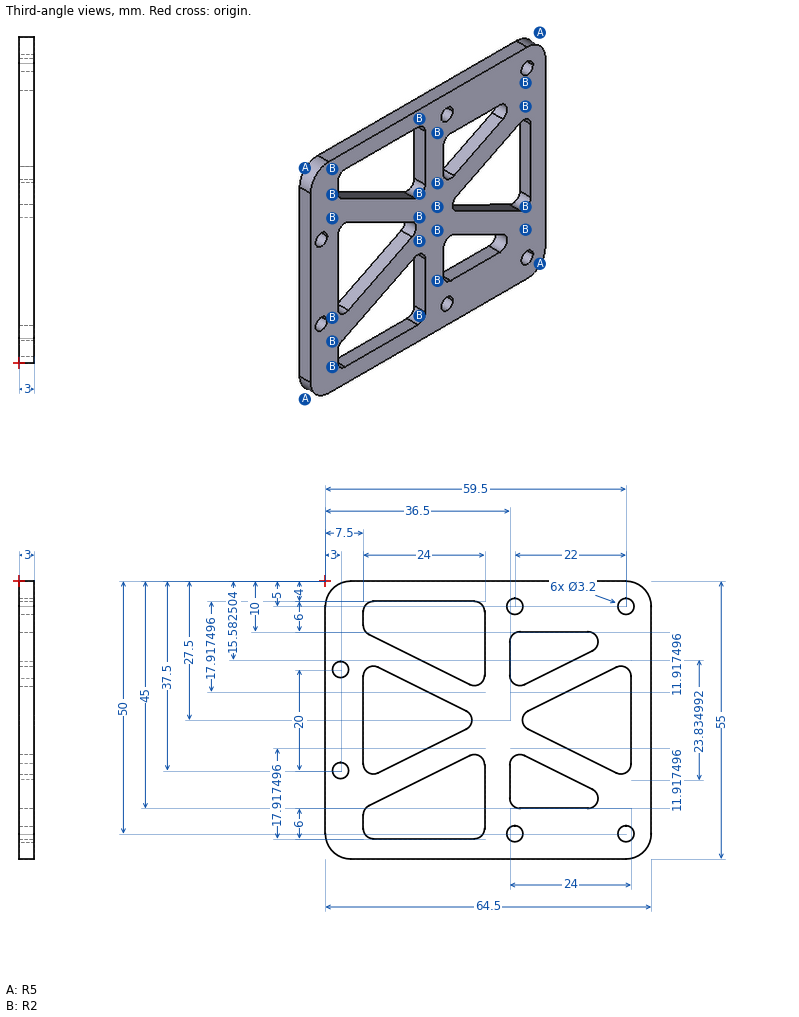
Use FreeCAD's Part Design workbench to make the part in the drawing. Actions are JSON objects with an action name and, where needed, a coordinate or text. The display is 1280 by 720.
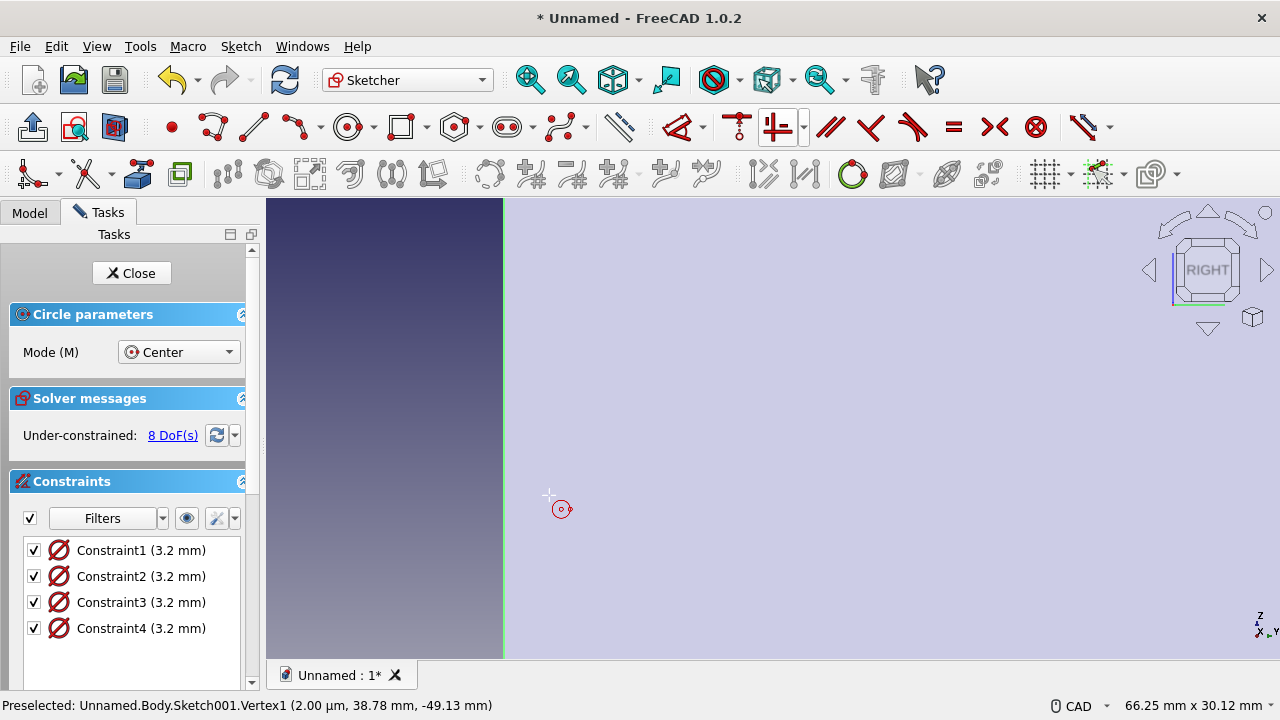
{"action": "left_click", "coordinate": [550, 494]}
{"action": "mouse_move", "coordinate": [567, 477]}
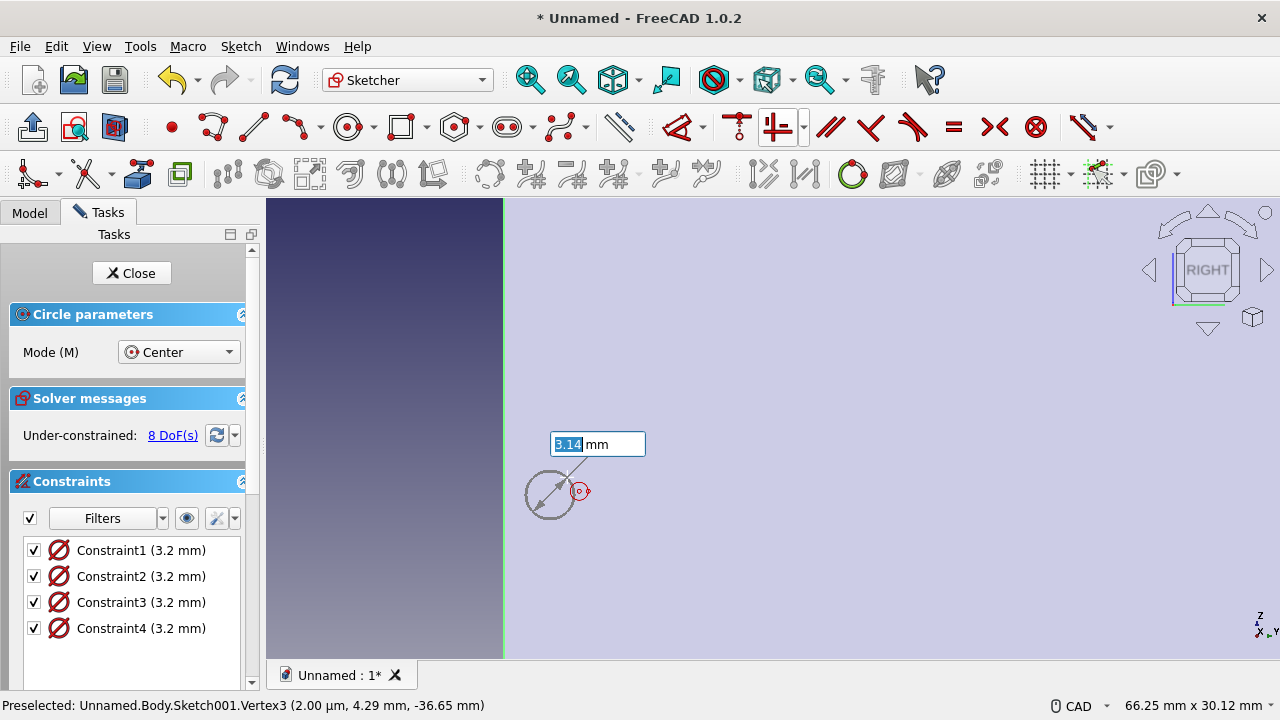
{"action": "type", "text": "3.2"}
{"action": "key", "text": "Return"}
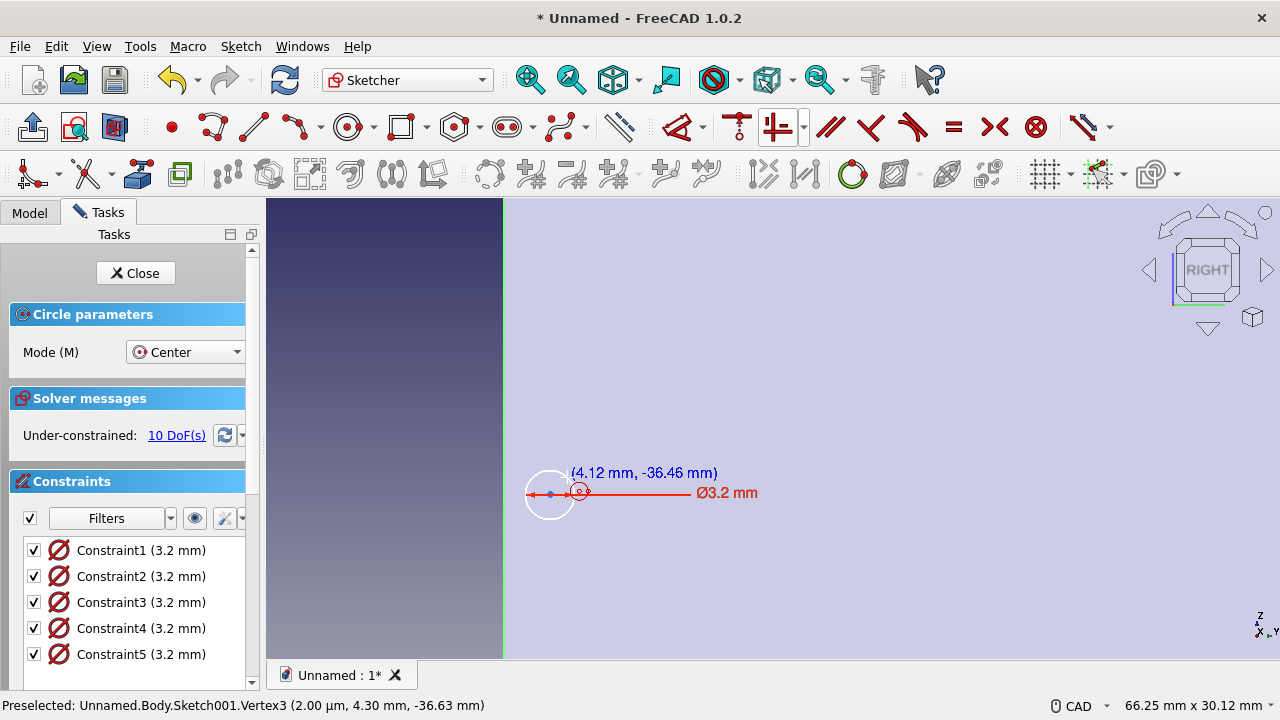
{"action": "scroll", "coordinate": [549, 495], "scroll_direction": "down", "scroll_amount": 5}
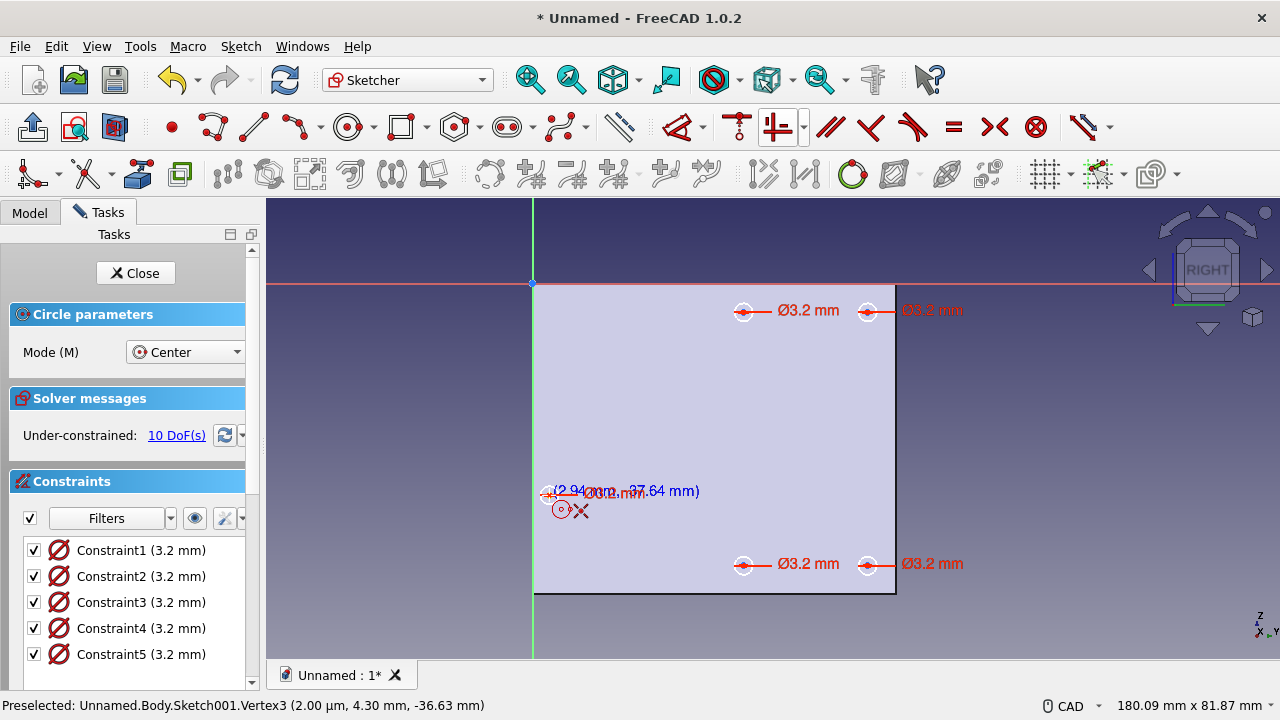
{"action": "scroll", "coordinate": [549, 382], "scroll_direction": "up", "scroll_amount": 5}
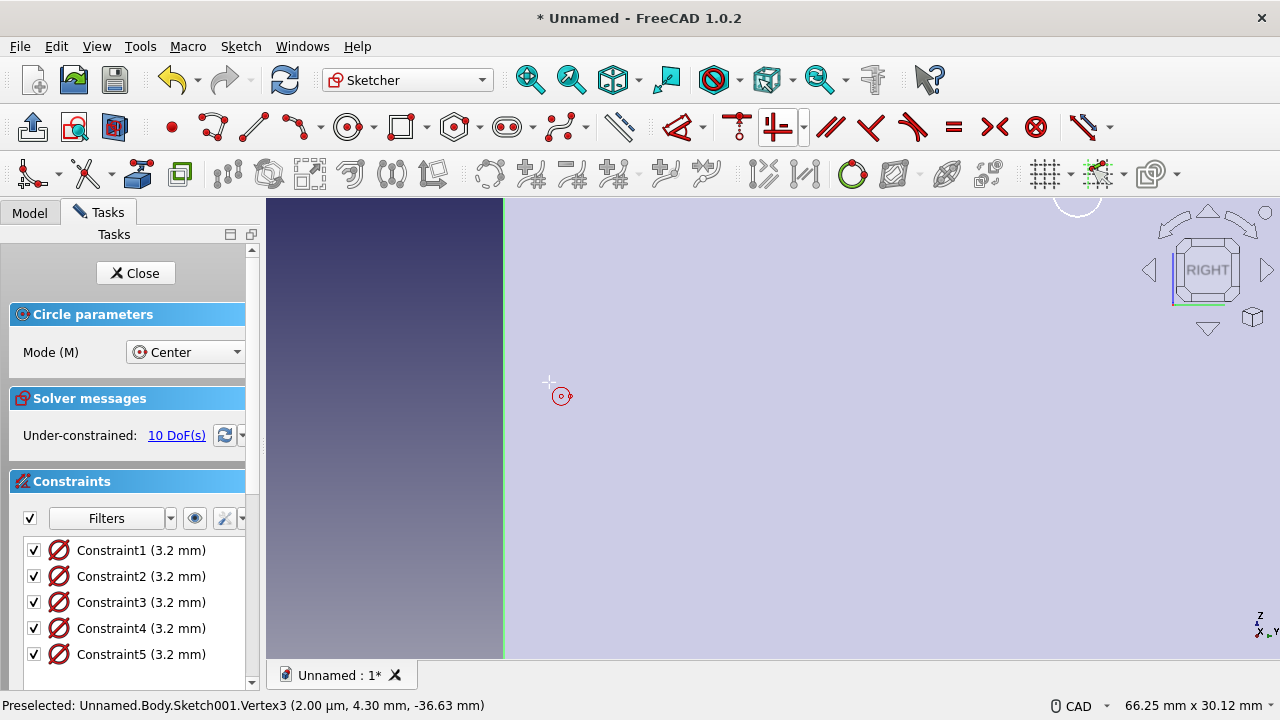
{"action": "left_click", "coordinate": [550, 382]}
{"action": "mouse_move", "coordinate": [567, 365]}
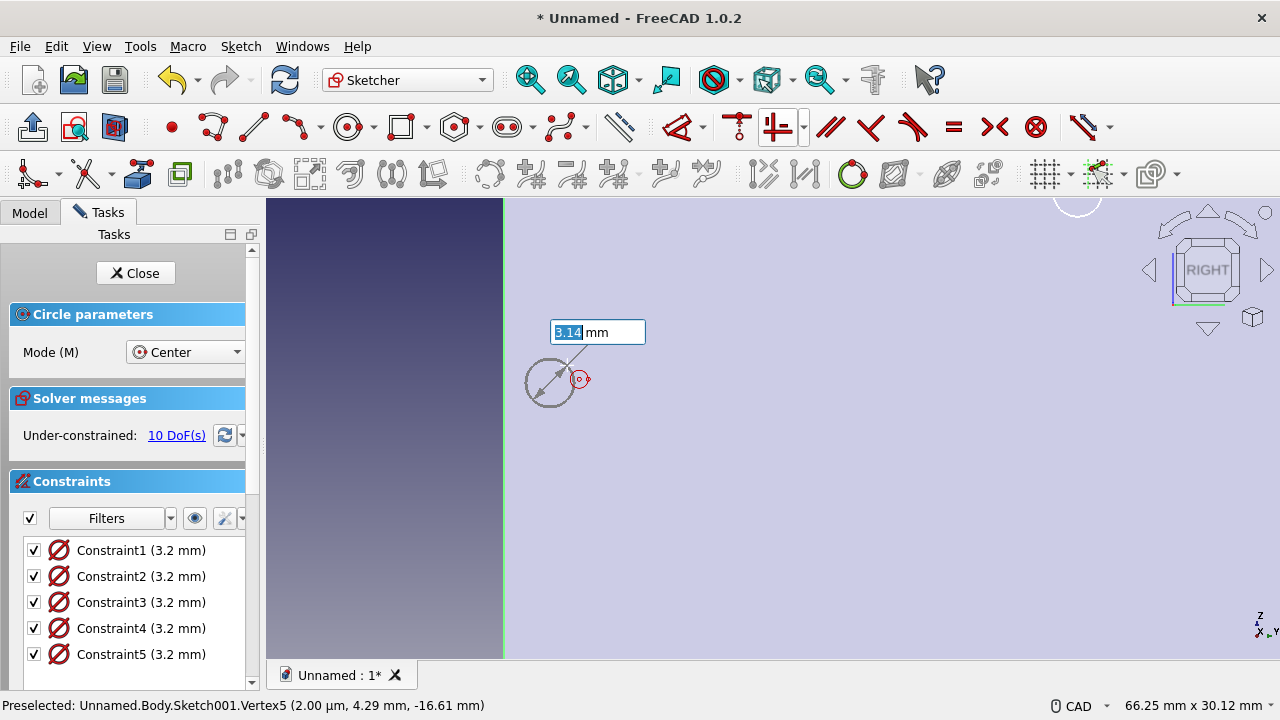
{"action": "type", "text": "3.2"}
{"action": "key", "text": "Return"}
{"action": "key", "text": "Escape"}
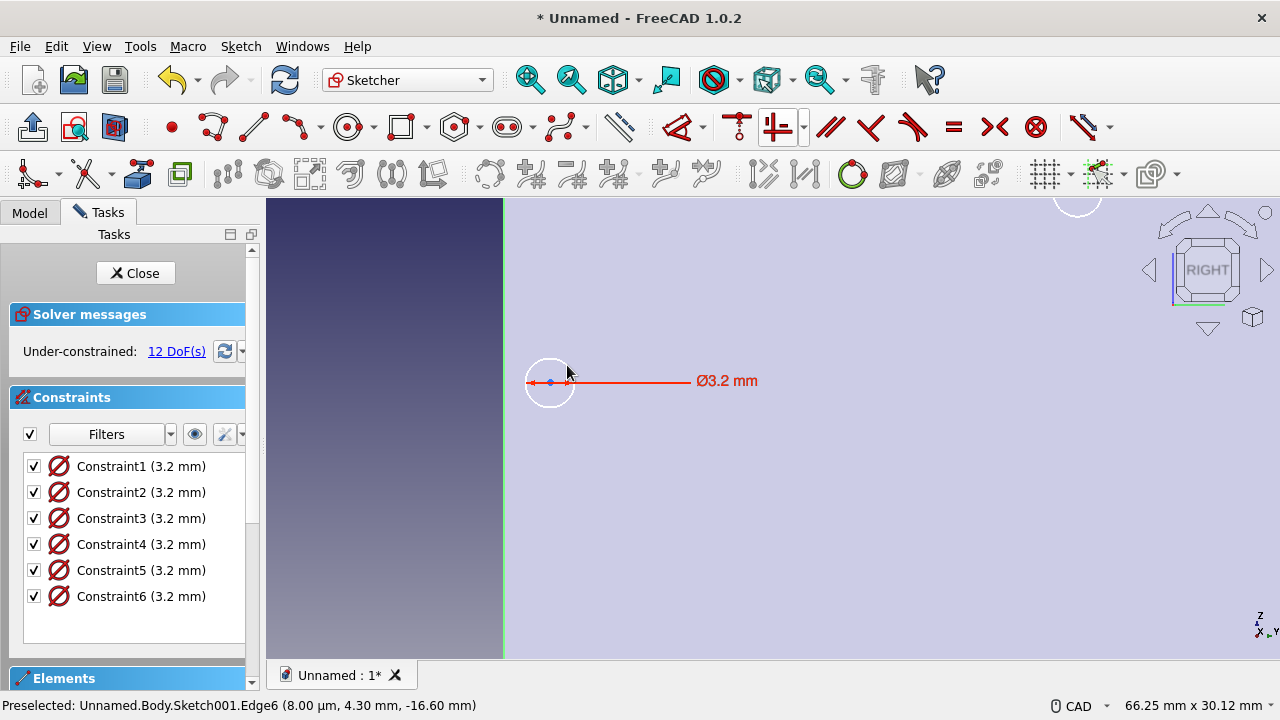
{"action": "scroll", "coordinate": [549, 381], "scroll_direction": "down", "scroll_amount": 5}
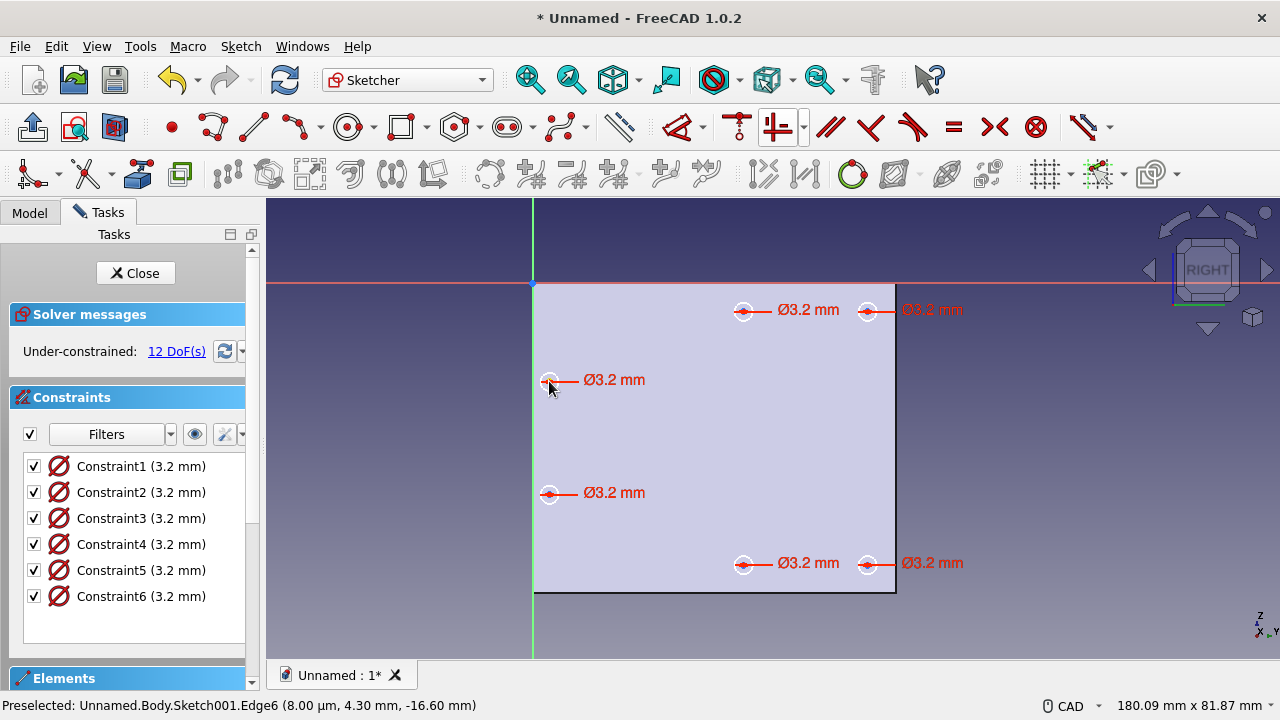
{"action": "left_click", "coordinate": [868, 312]}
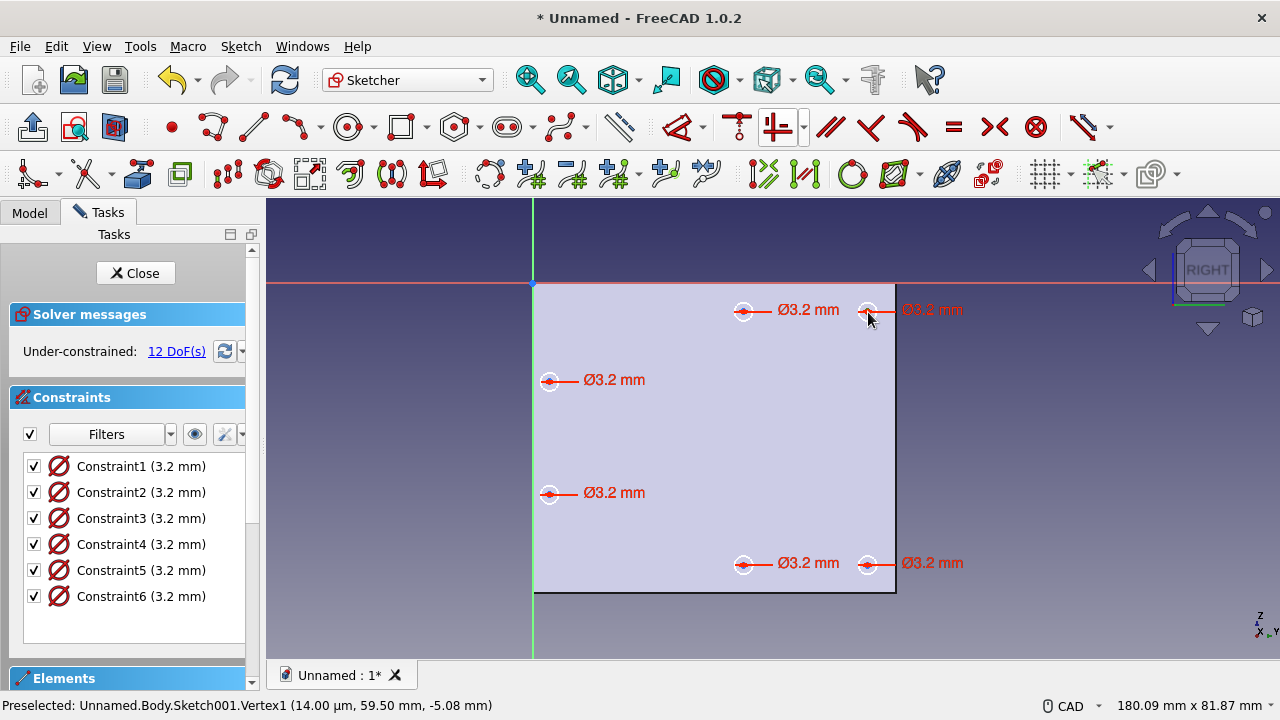
{"action": "left_click", "coordinate": [744, 312]}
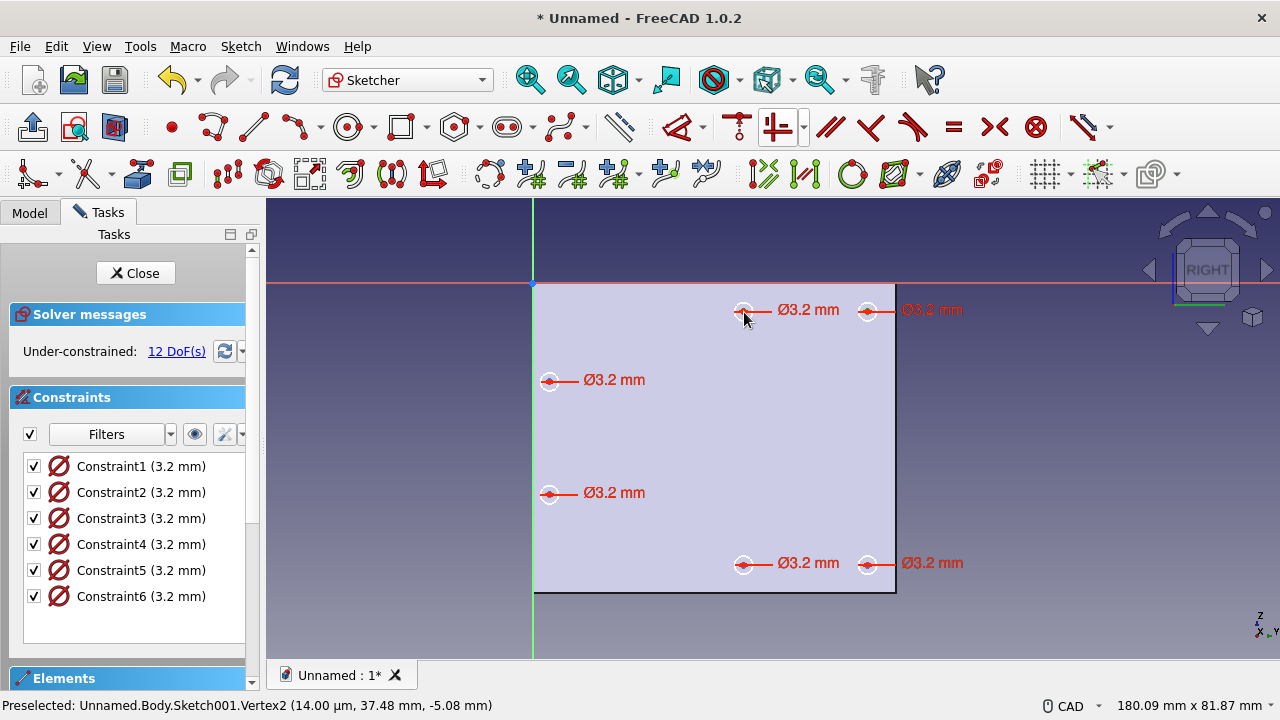
{"action": "key", "text": "h"}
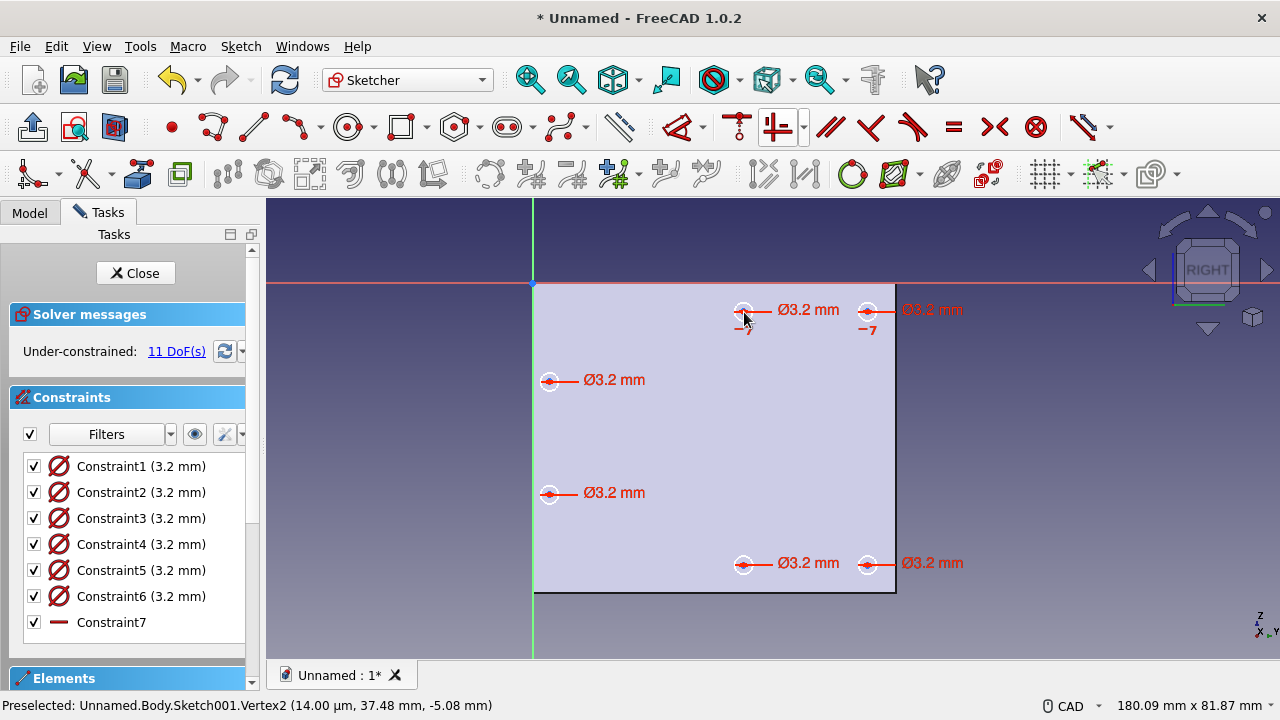
{"action": "left_click", "coordinate": [868, 312]}